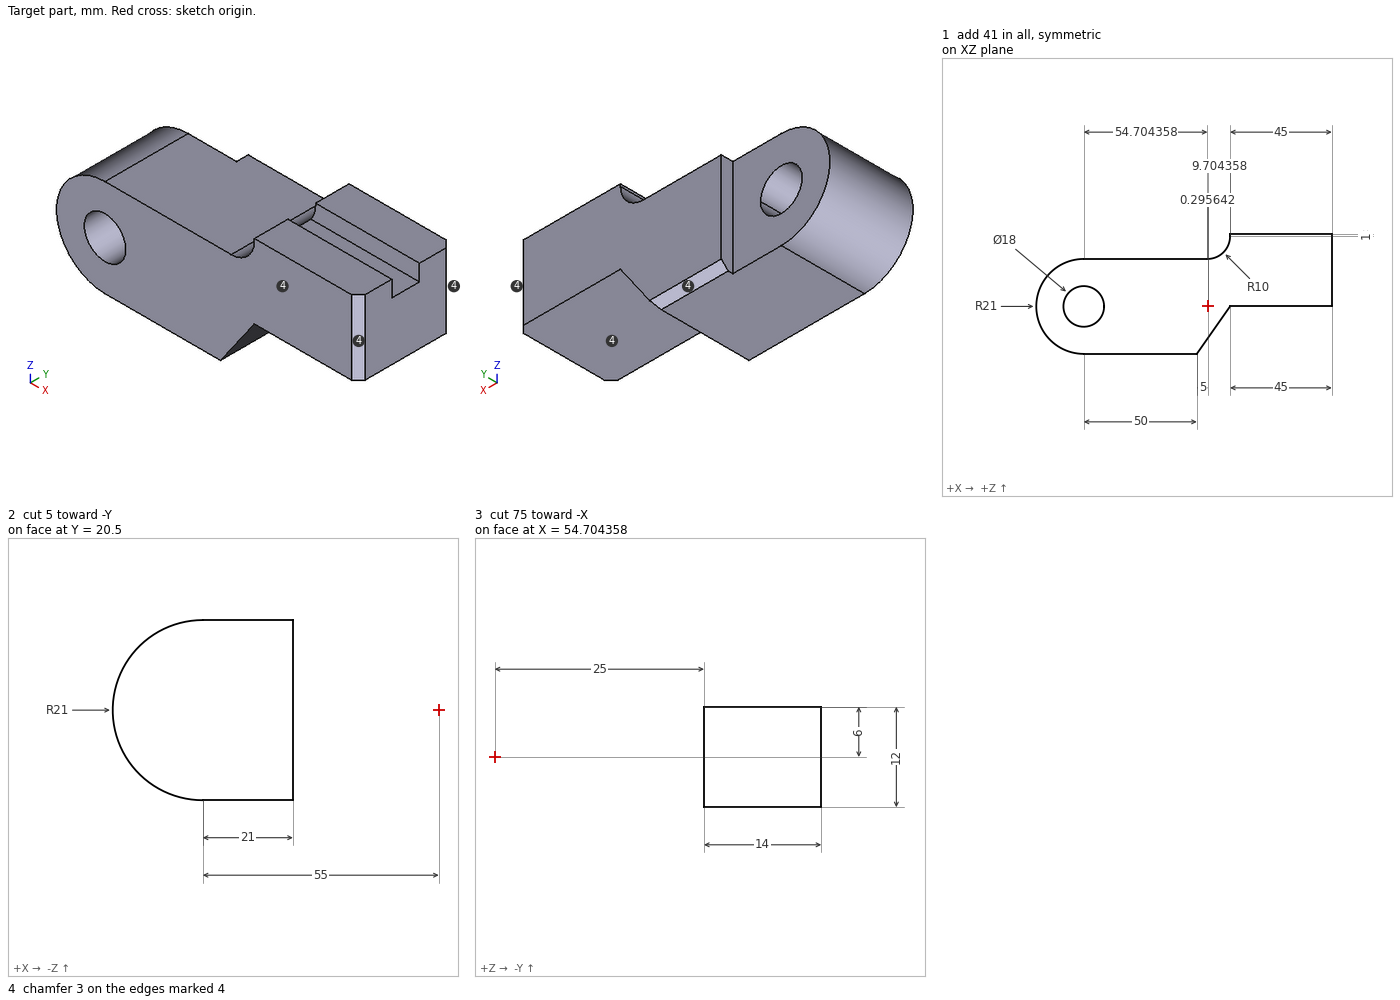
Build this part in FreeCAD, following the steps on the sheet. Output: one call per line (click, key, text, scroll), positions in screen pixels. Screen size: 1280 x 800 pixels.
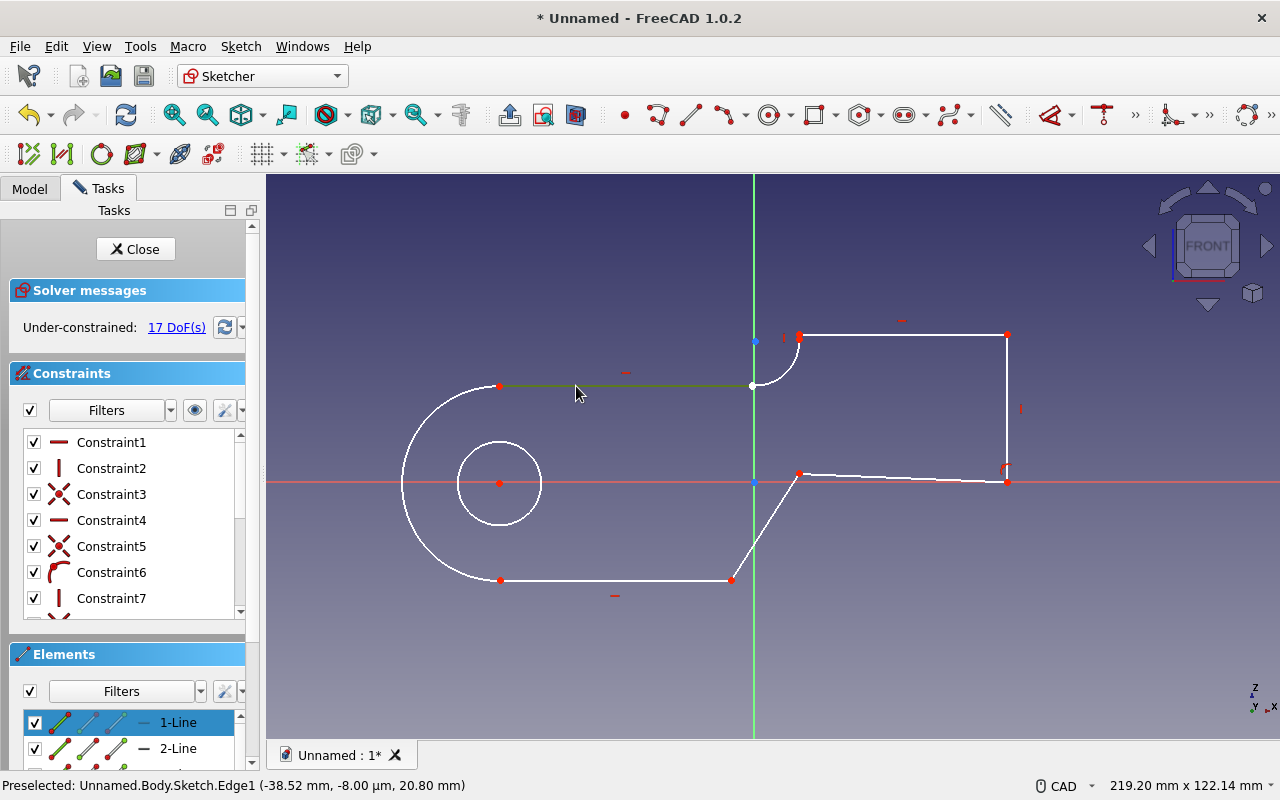
click(774, 381)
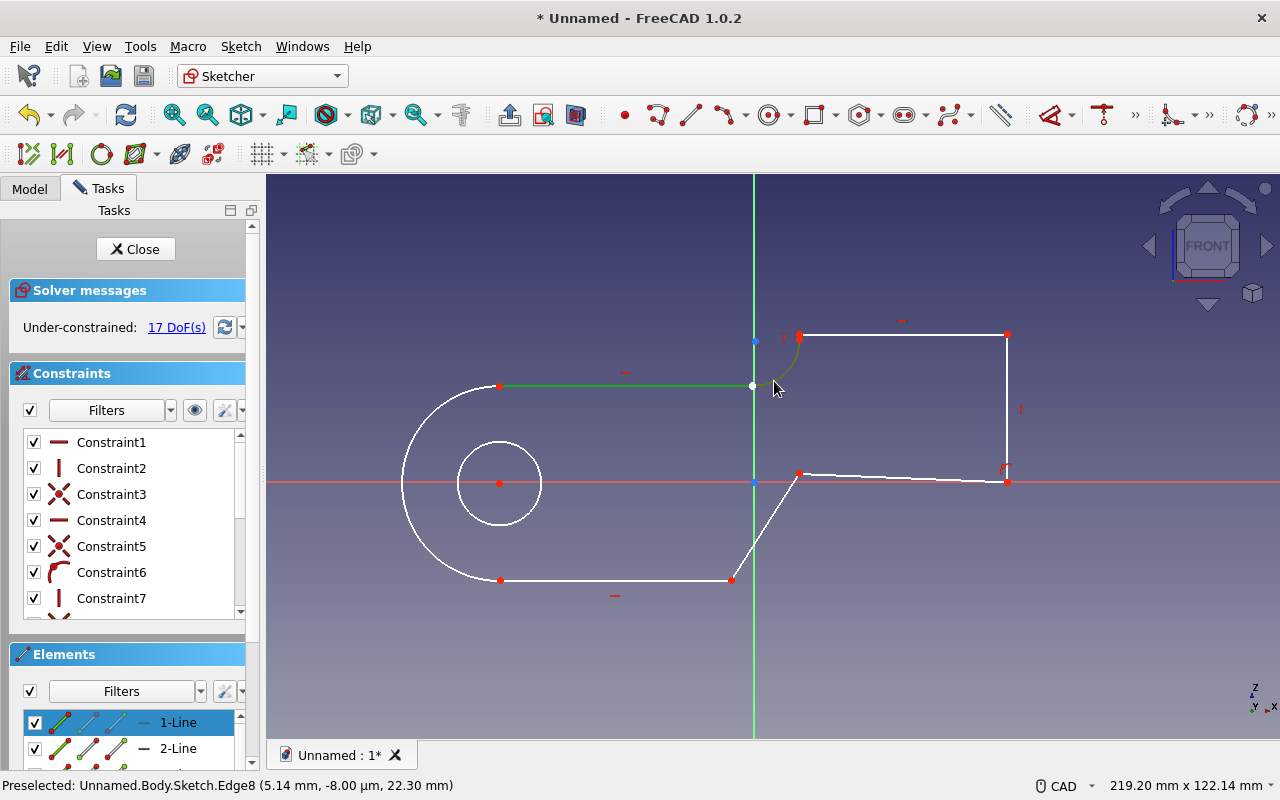
key(t)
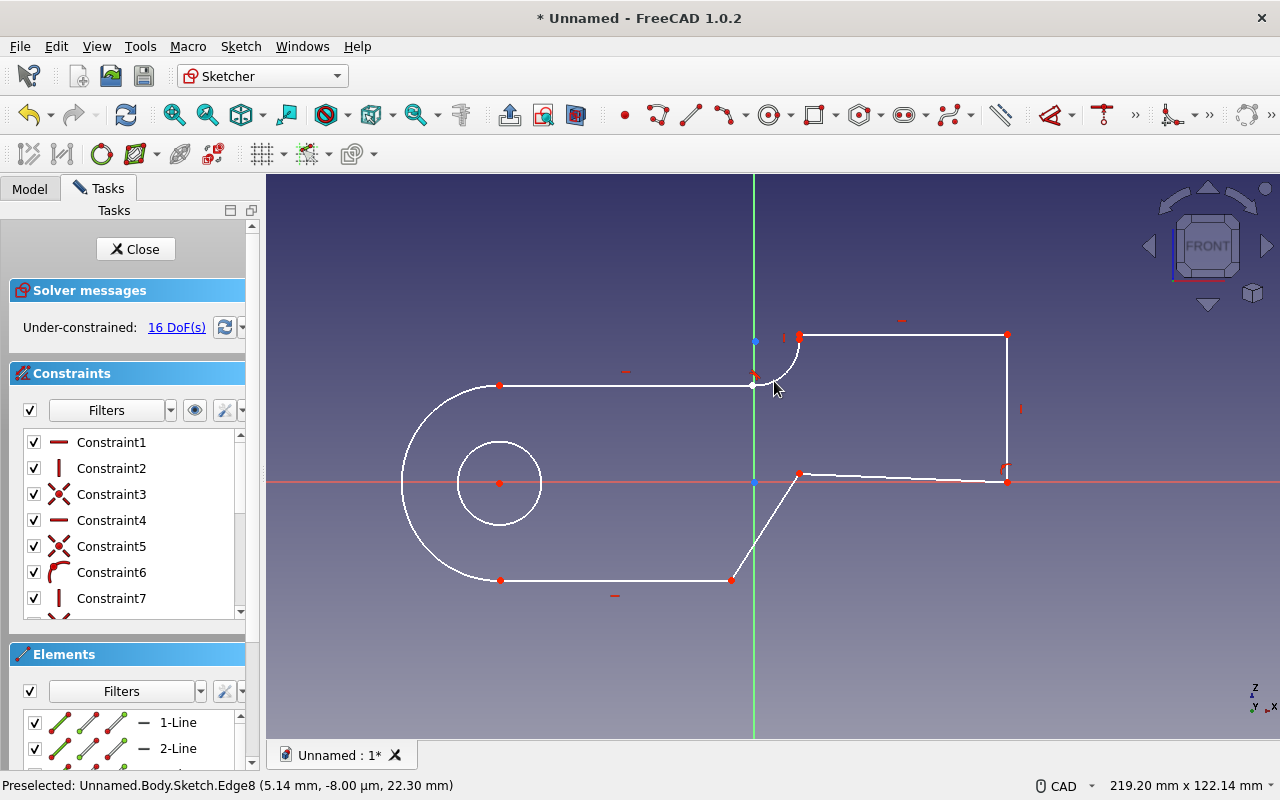
click(576, 386)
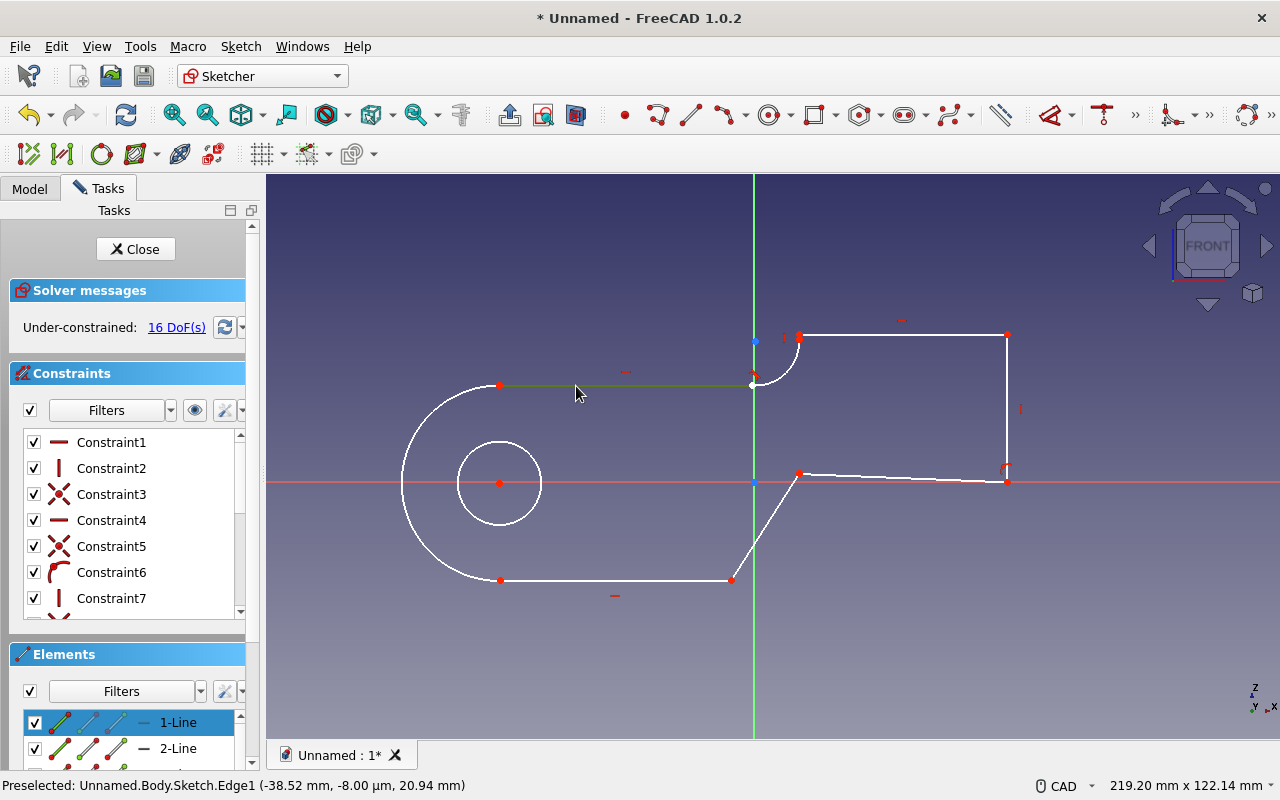
click(420, 426)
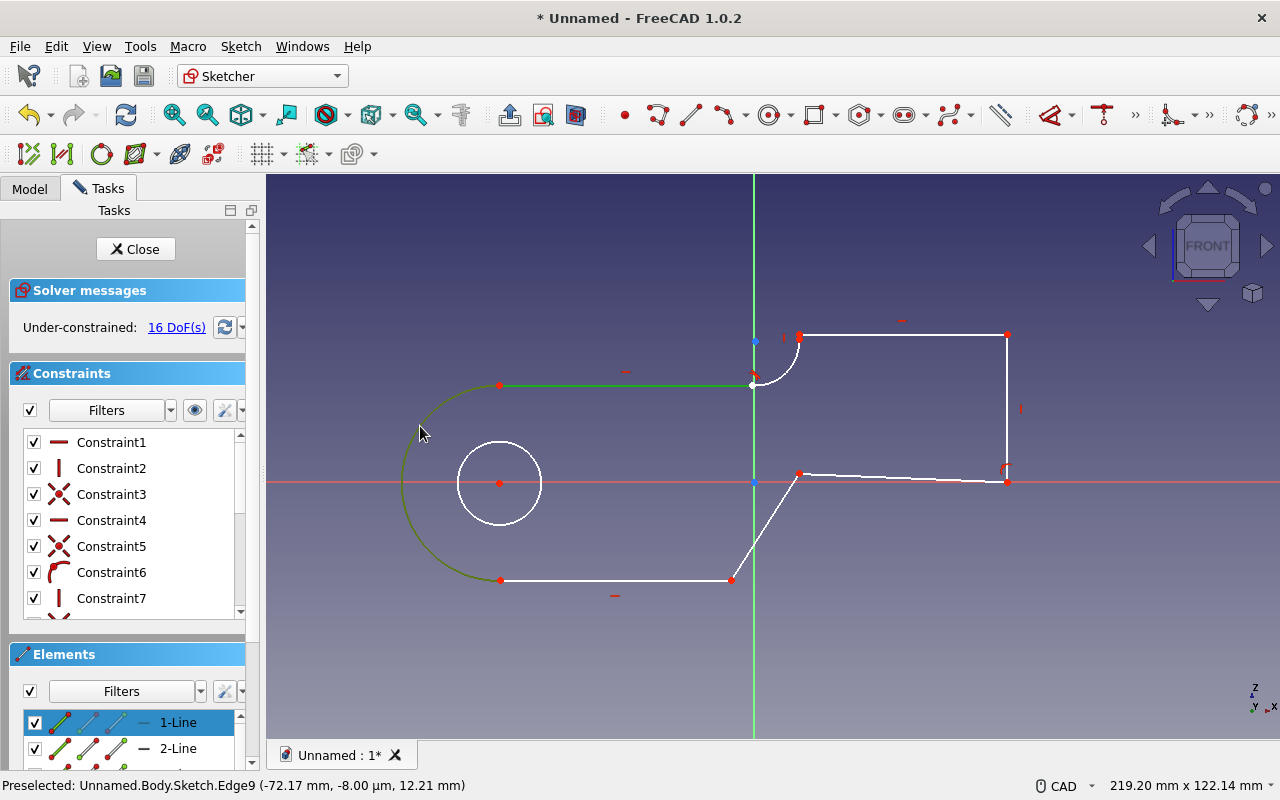
key(t)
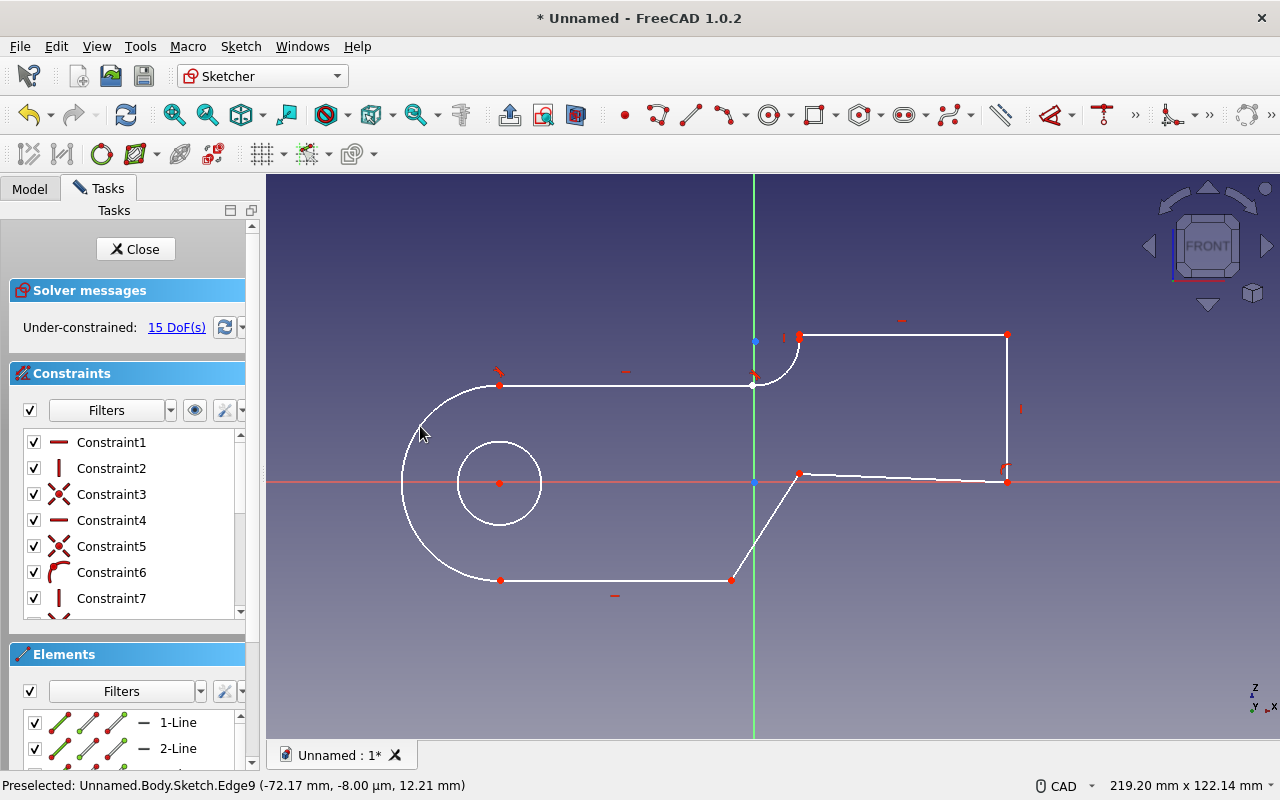
scroll(799, 337, up, 9)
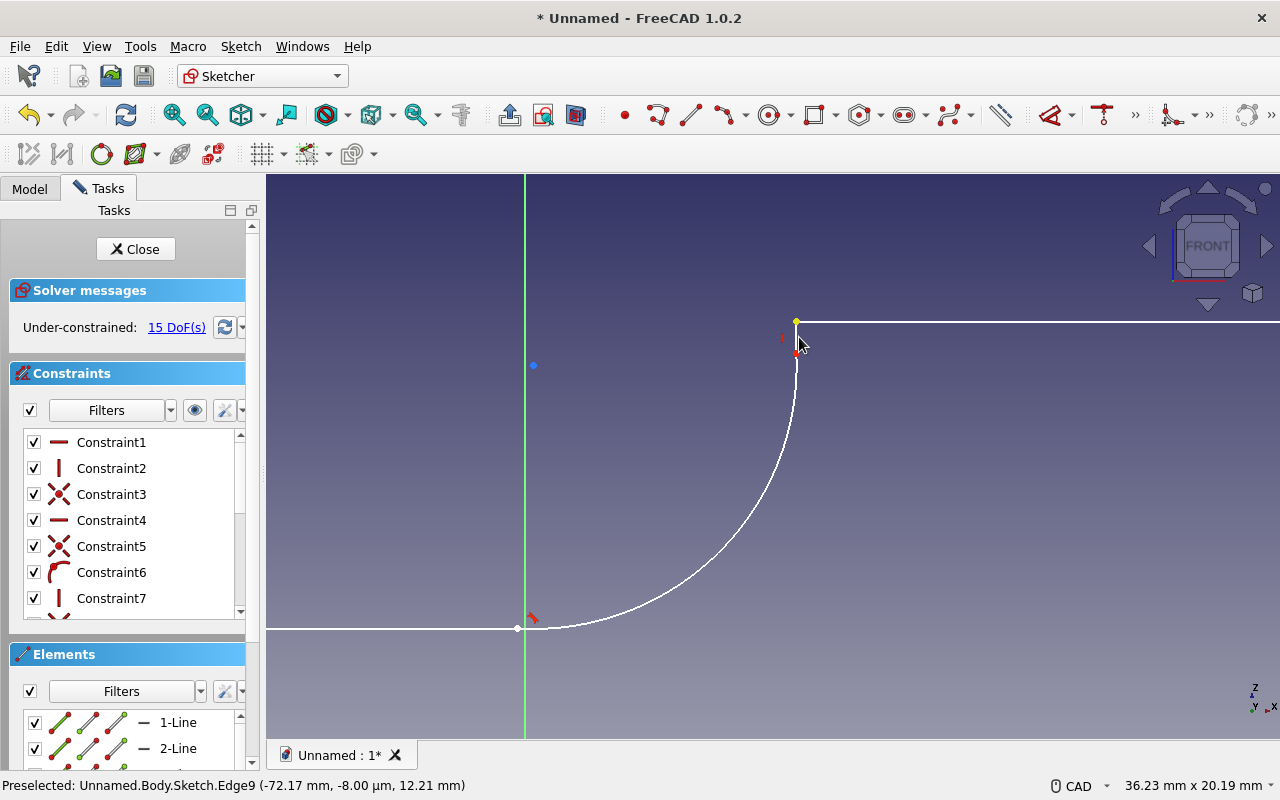
click(796, 338)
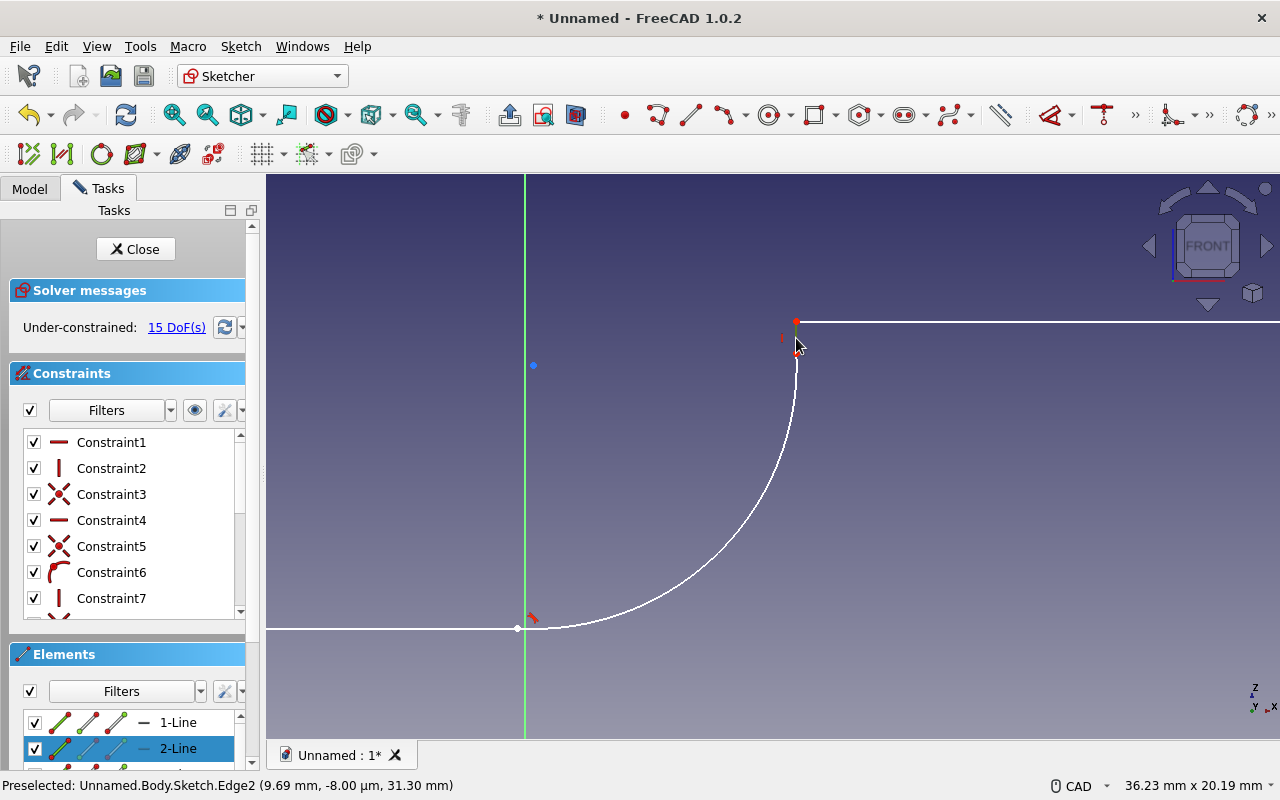
scroll(799, 337, down, 9)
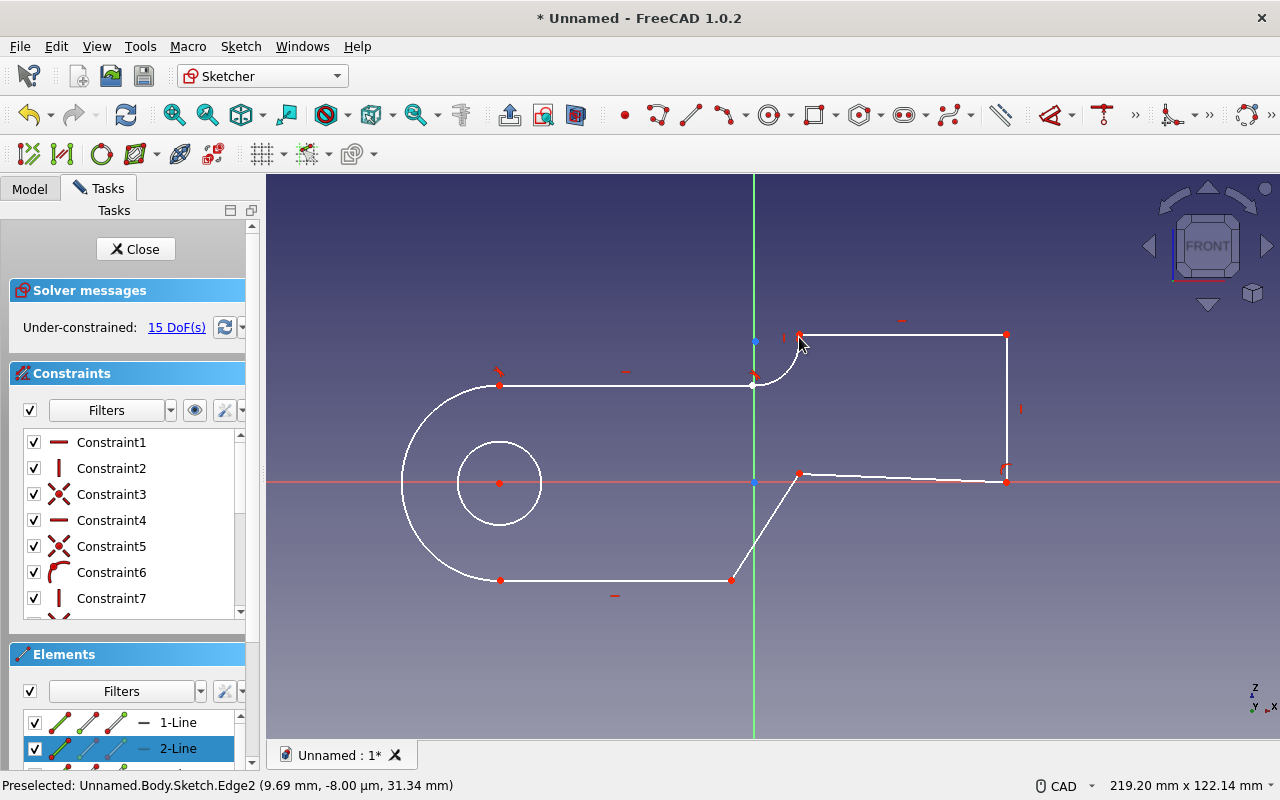
click(774, 381)